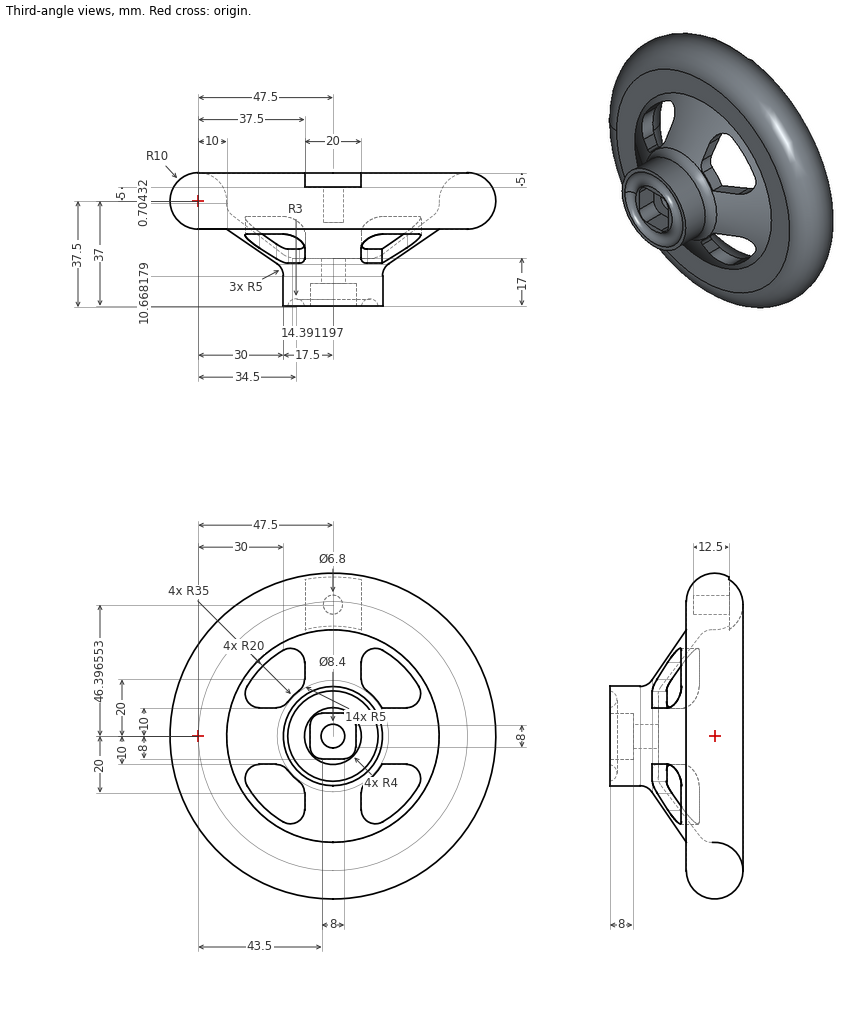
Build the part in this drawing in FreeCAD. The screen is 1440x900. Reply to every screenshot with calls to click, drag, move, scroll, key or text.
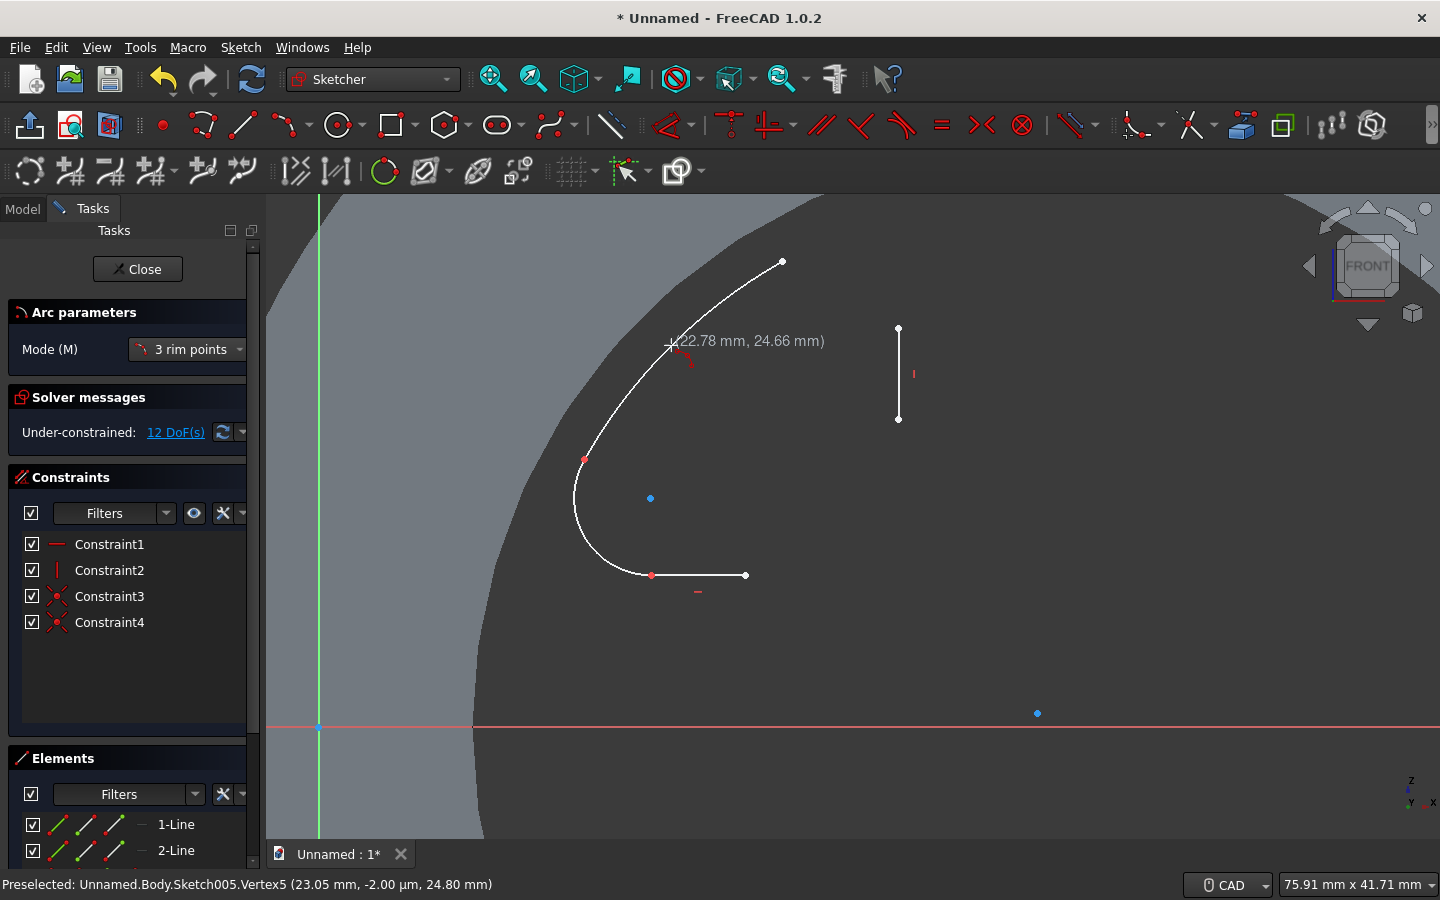
click(783, 261)
click(899, 328)
click(860, 259)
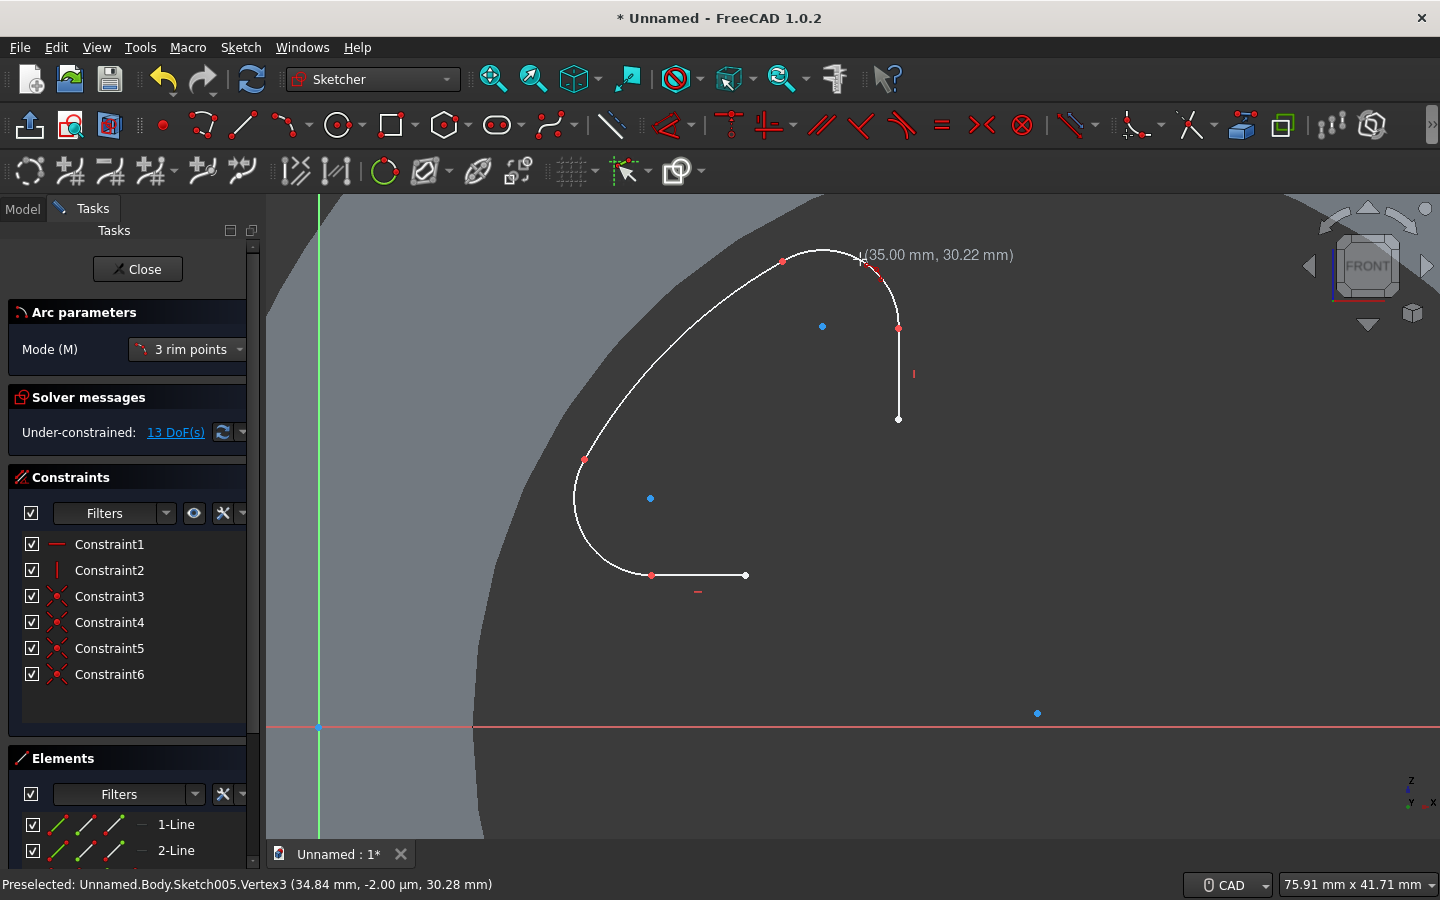
click(899, 419)
click(868, 480)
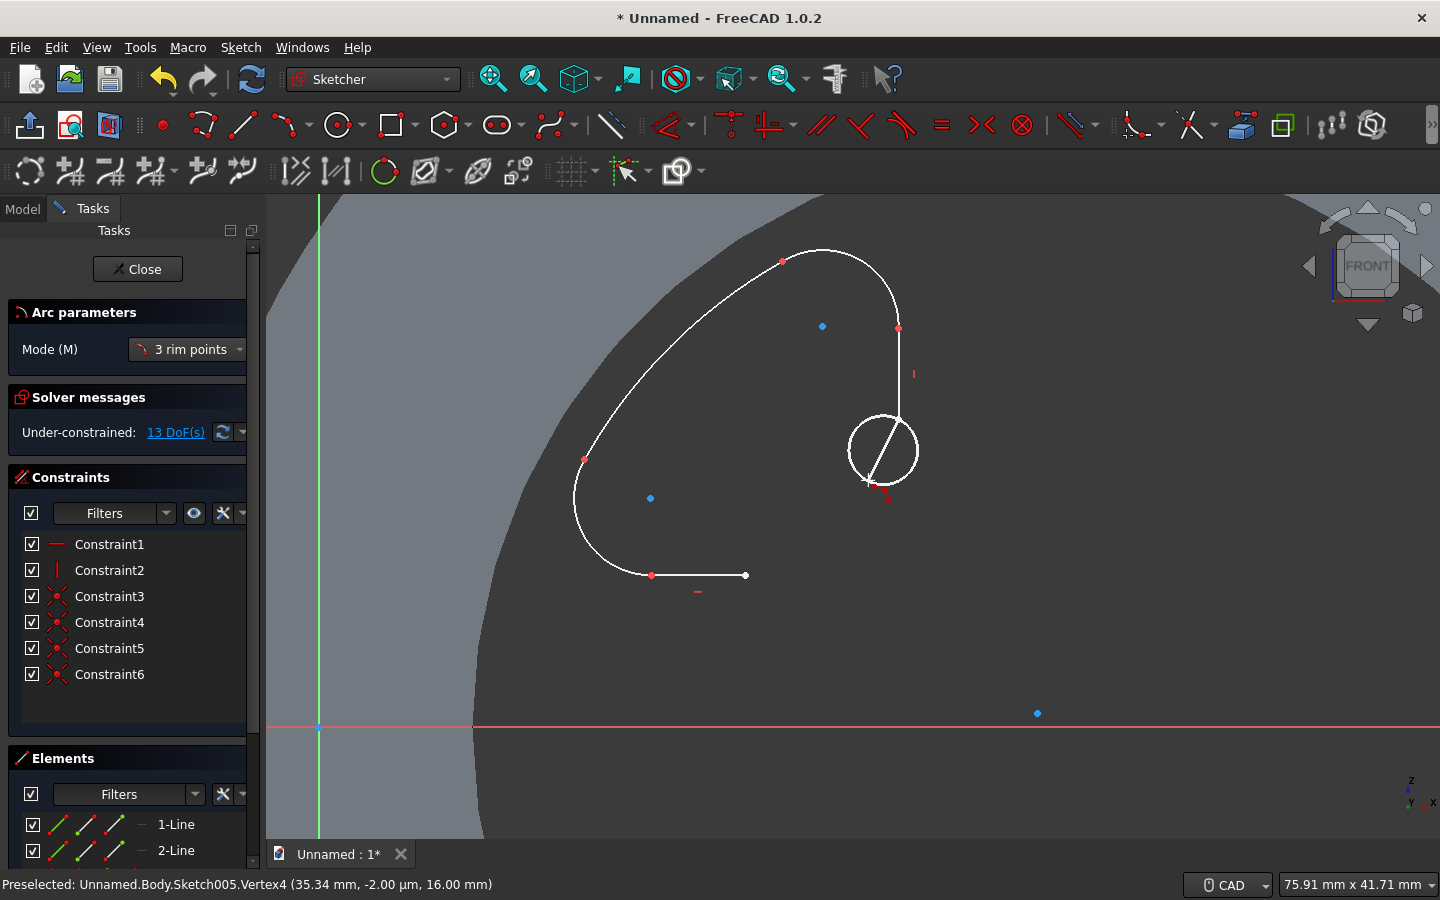
scroll(891, 453, up, 4)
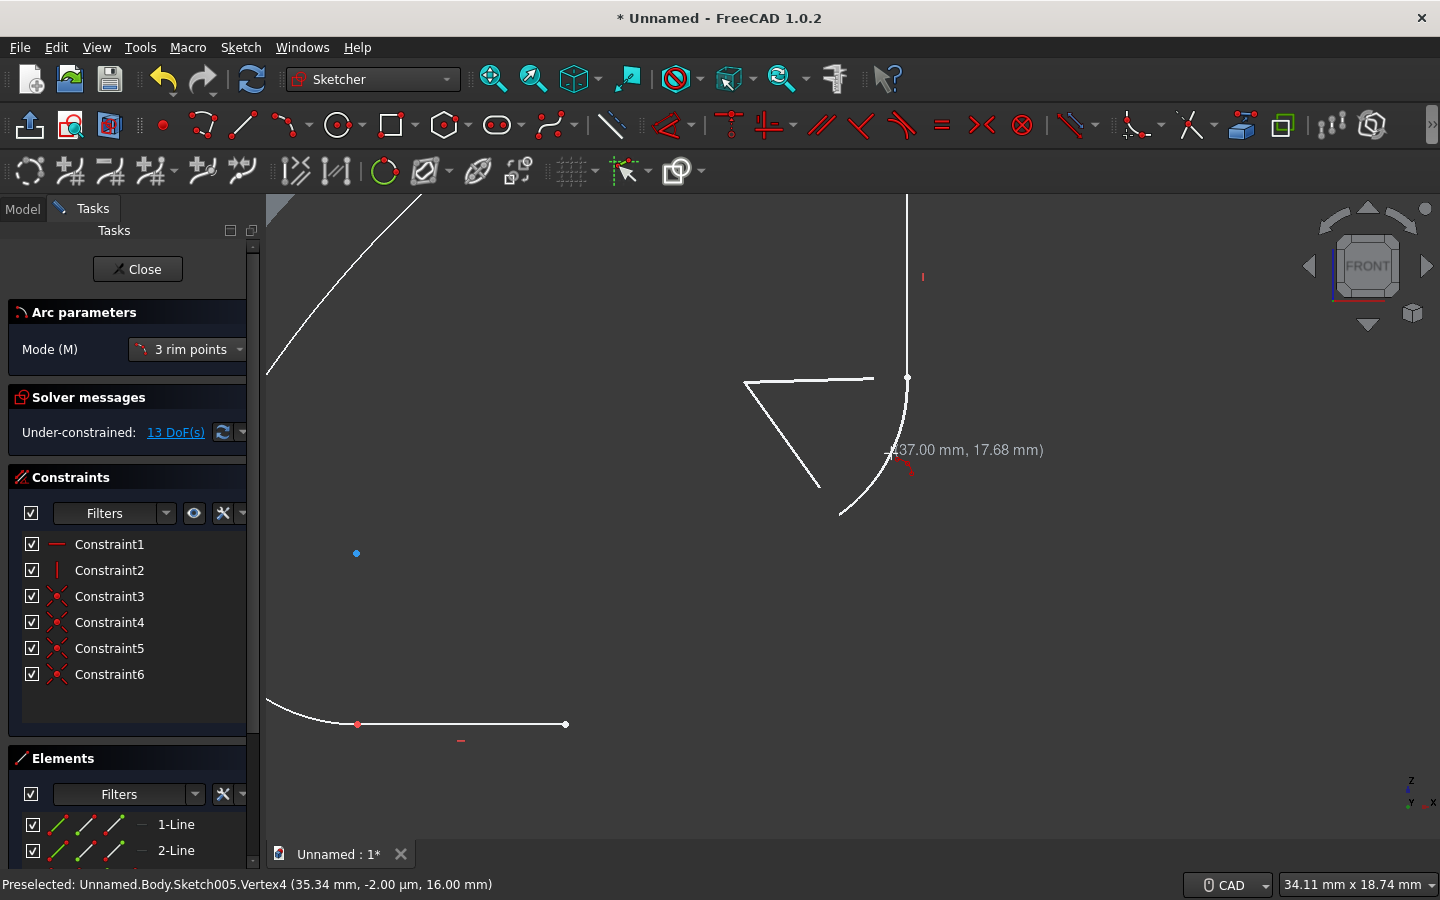
click(889, 452)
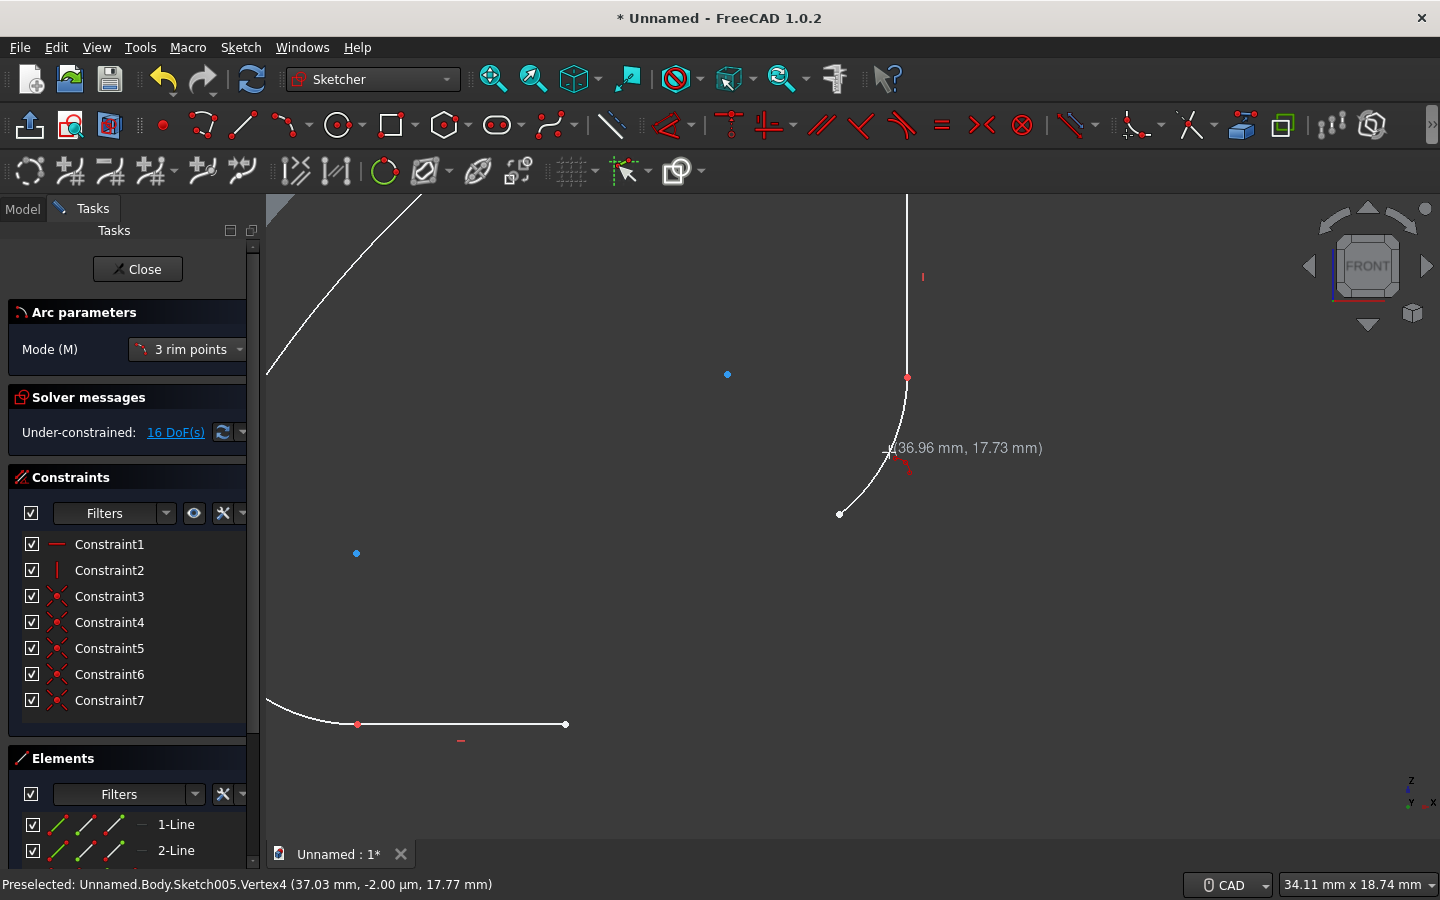
scroll(741, 378, down, 8)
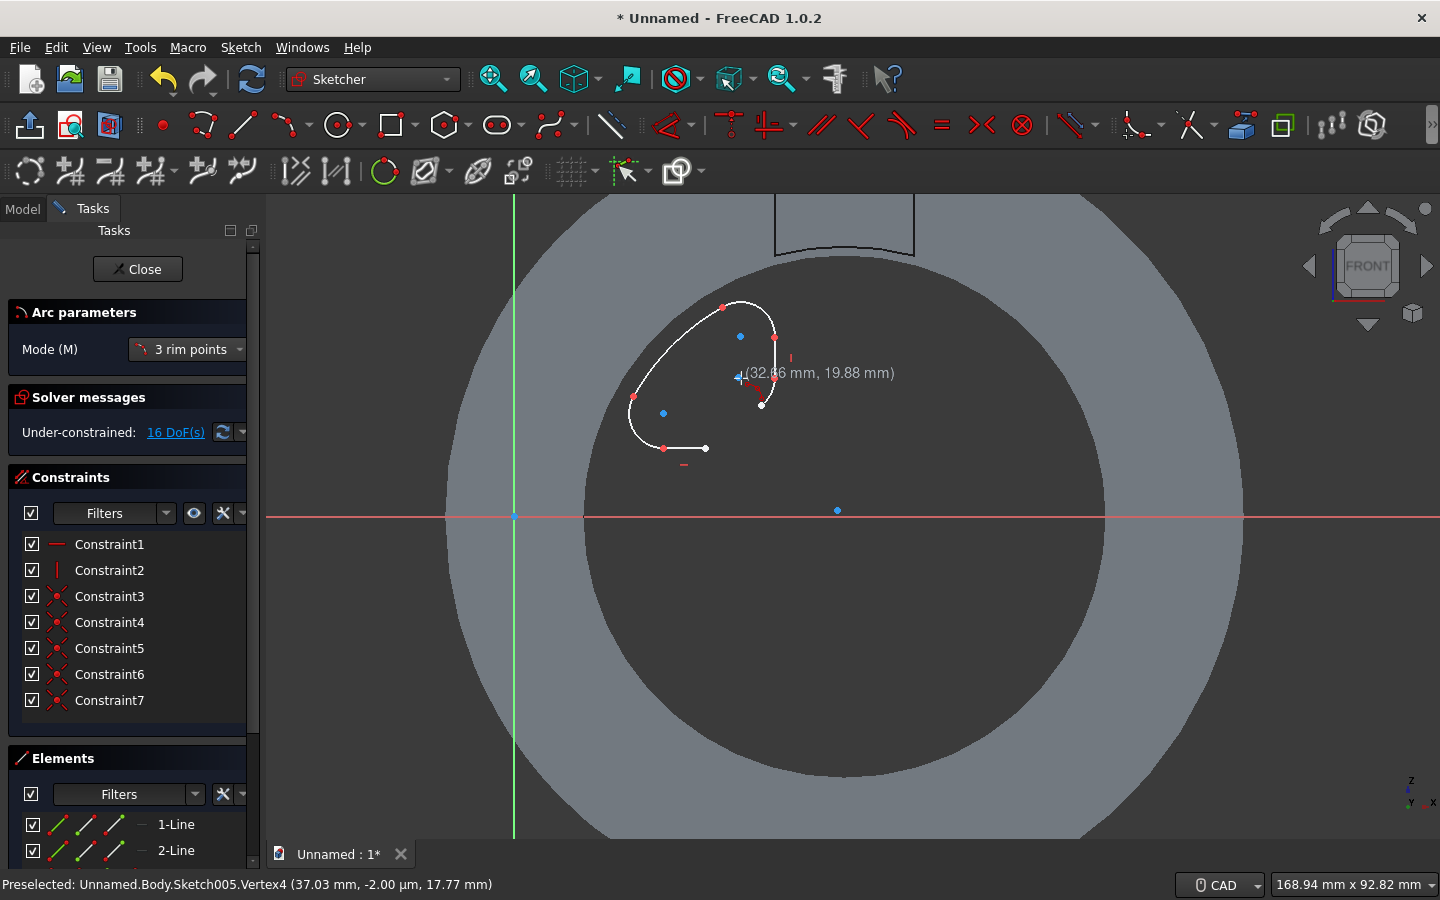
click(761, 406)
click(733, 433)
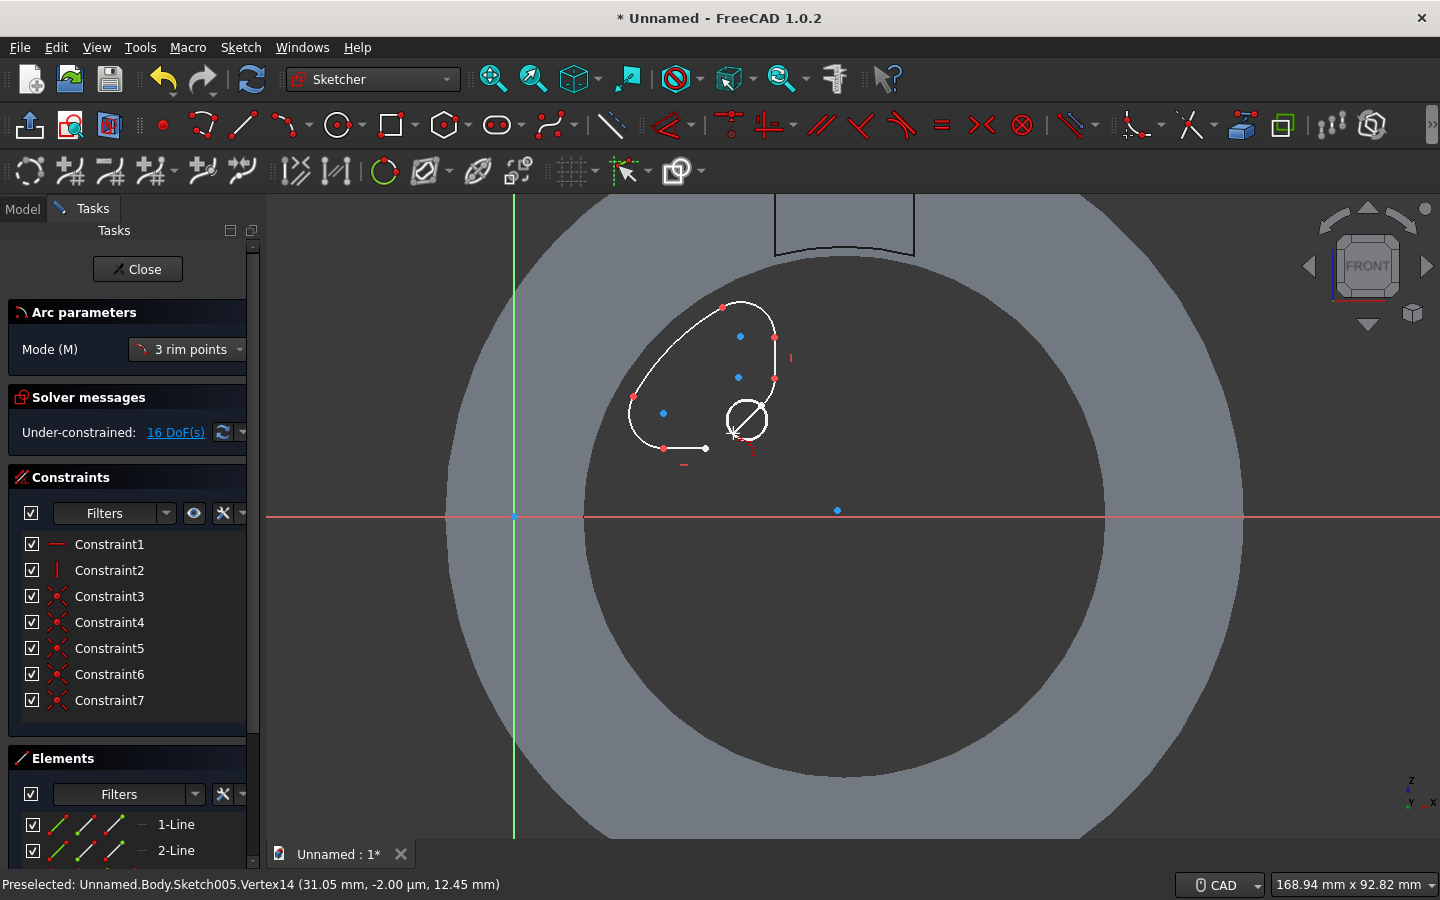
scroll(746, 418, up, 13)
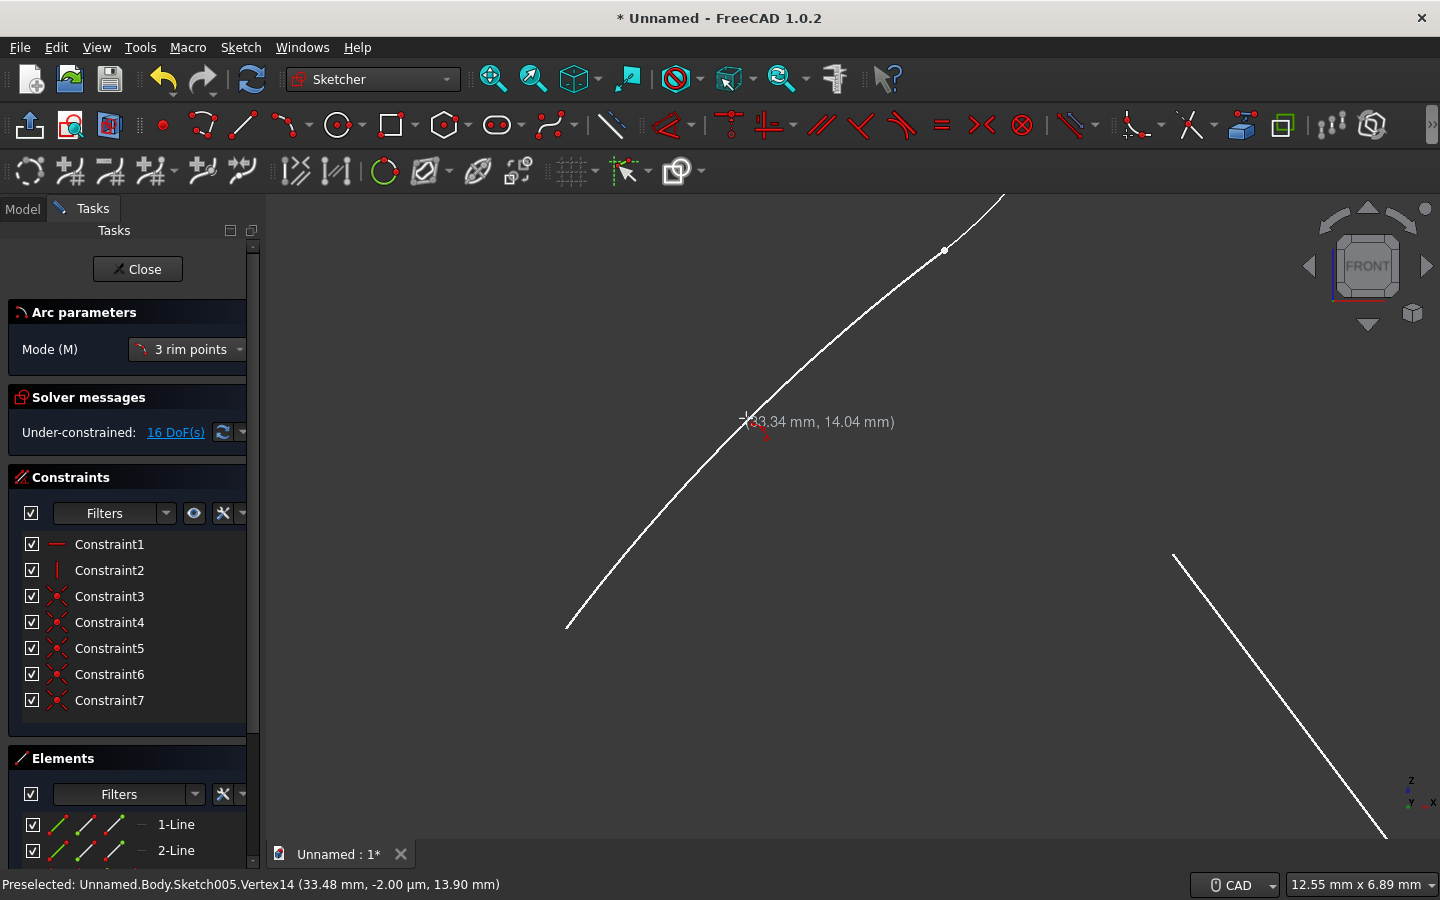
click(743, 418)